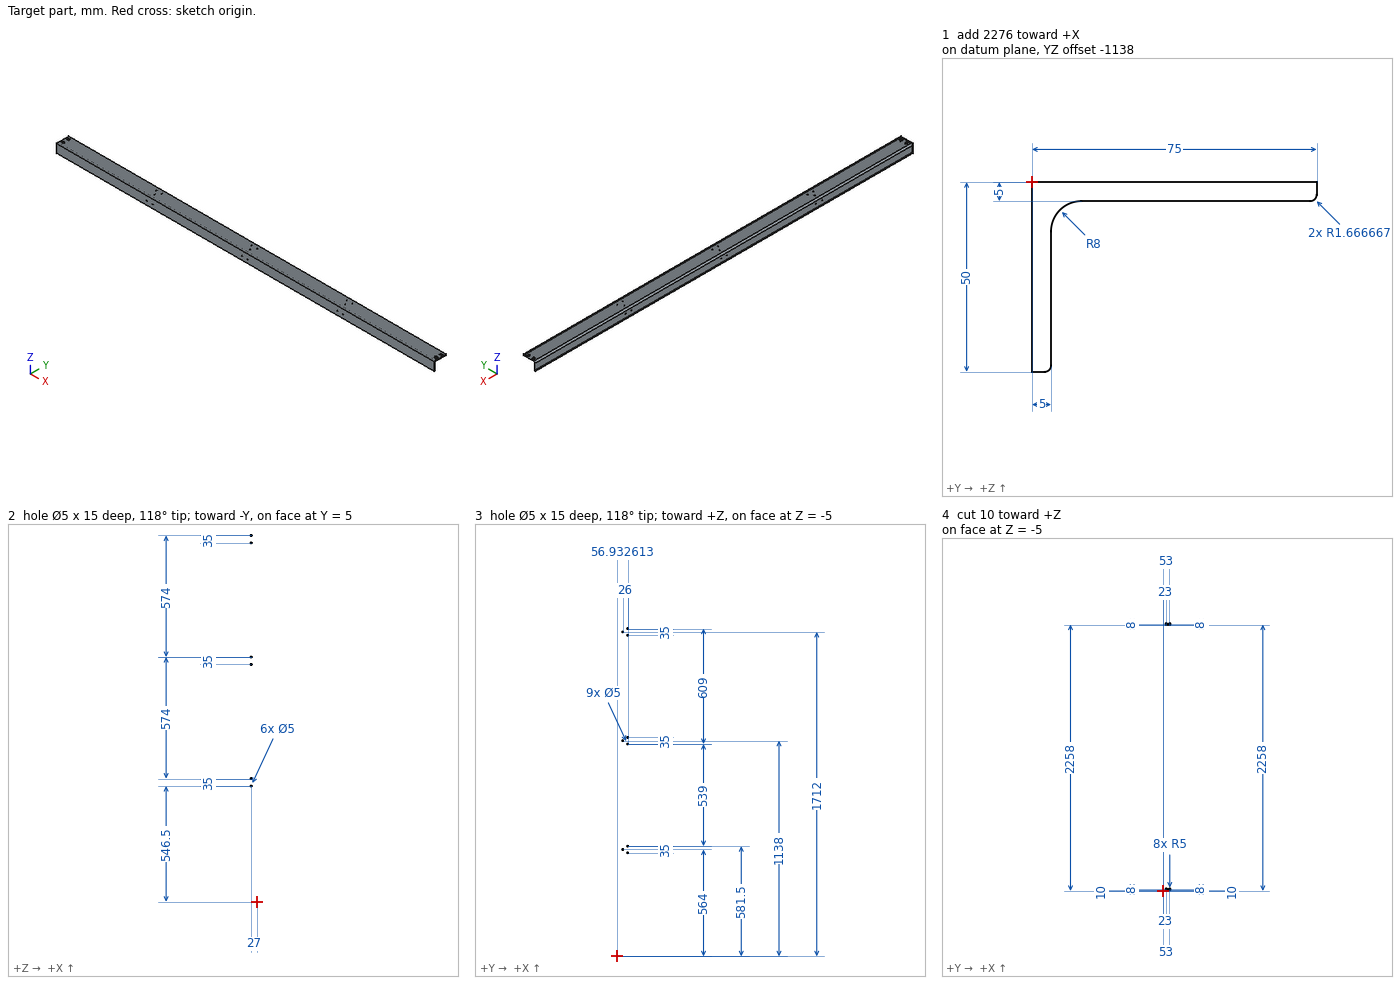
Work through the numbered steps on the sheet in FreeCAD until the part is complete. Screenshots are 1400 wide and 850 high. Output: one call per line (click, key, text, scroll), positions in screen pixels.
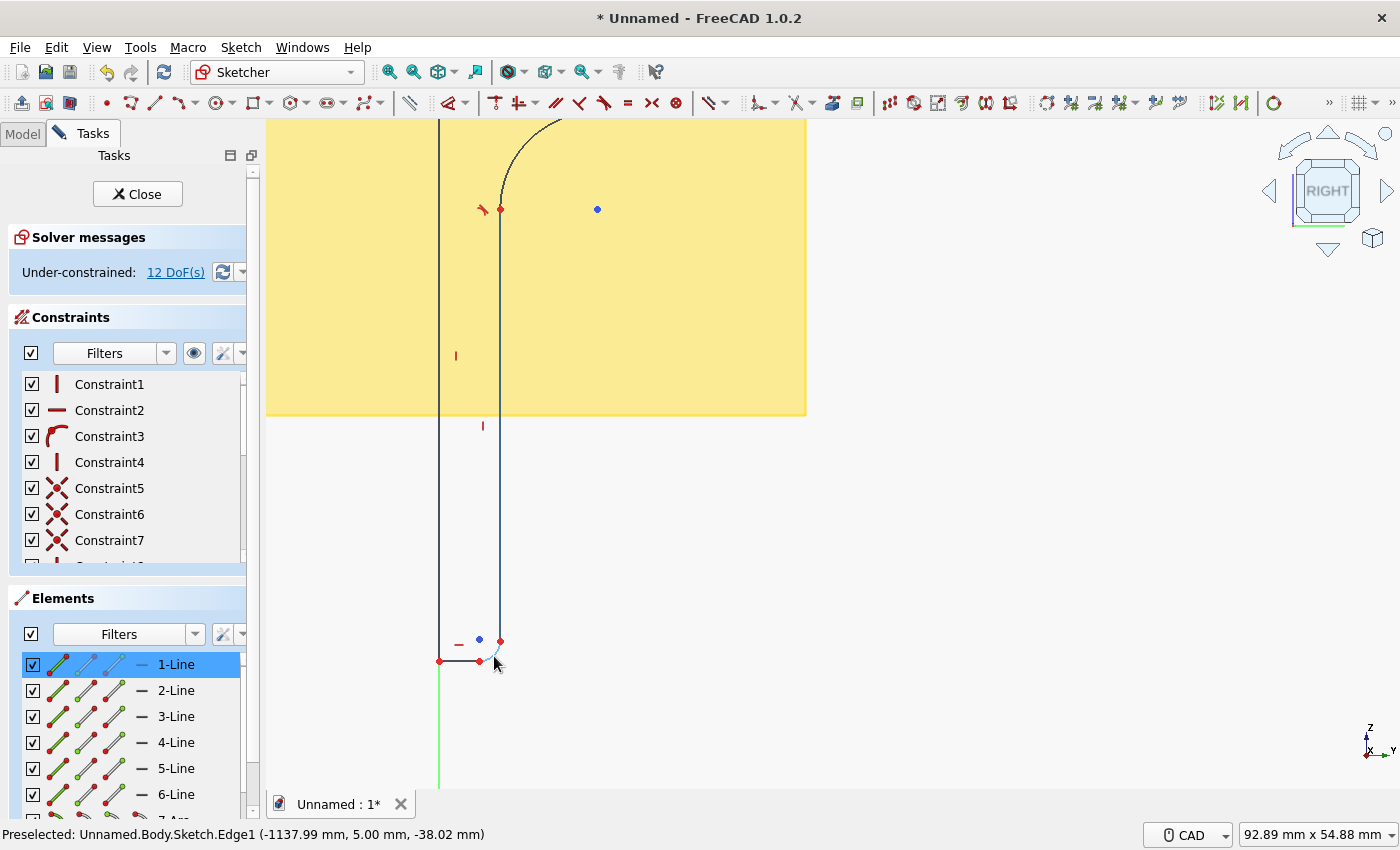
click(494, 656)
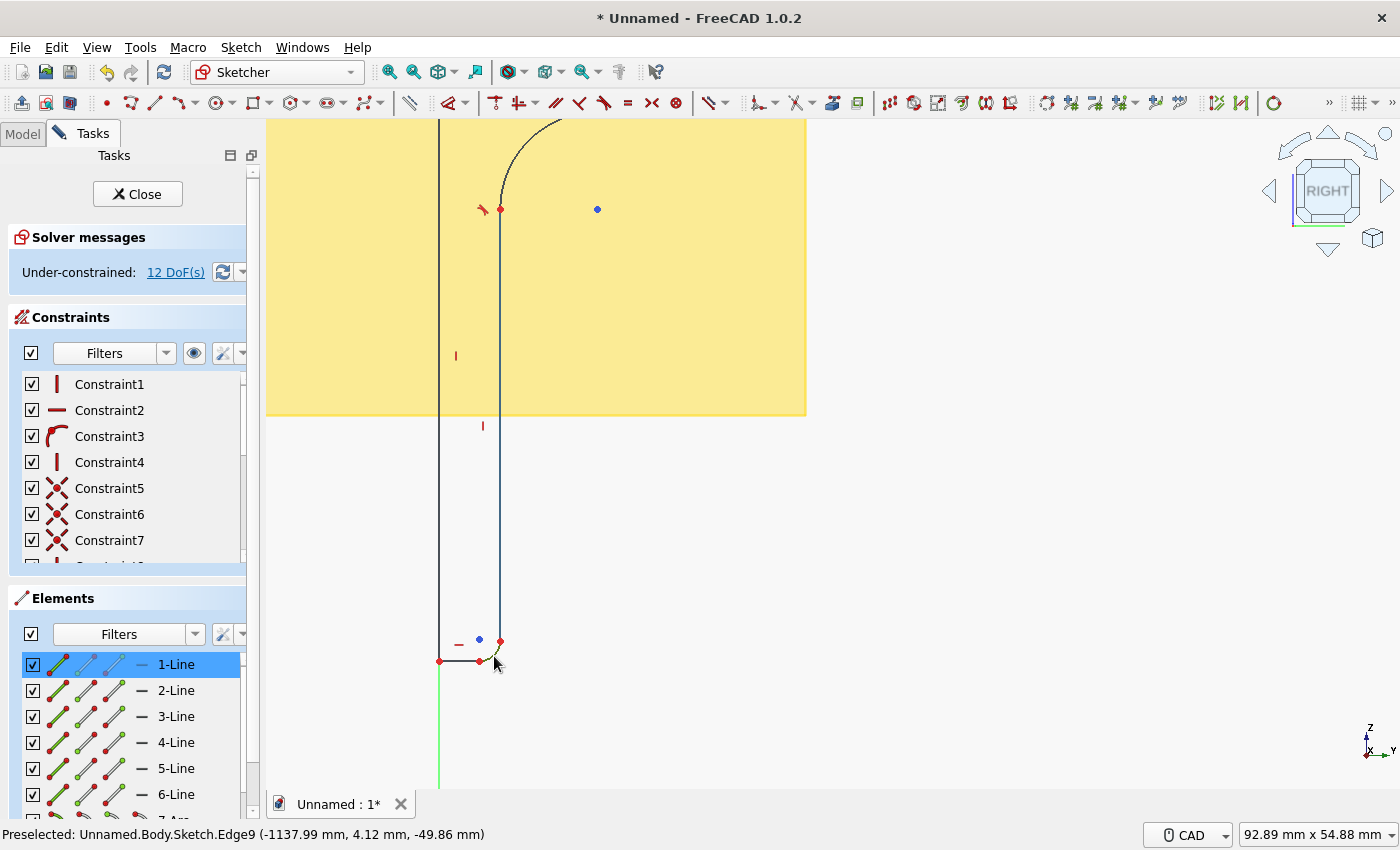
click(604, 104)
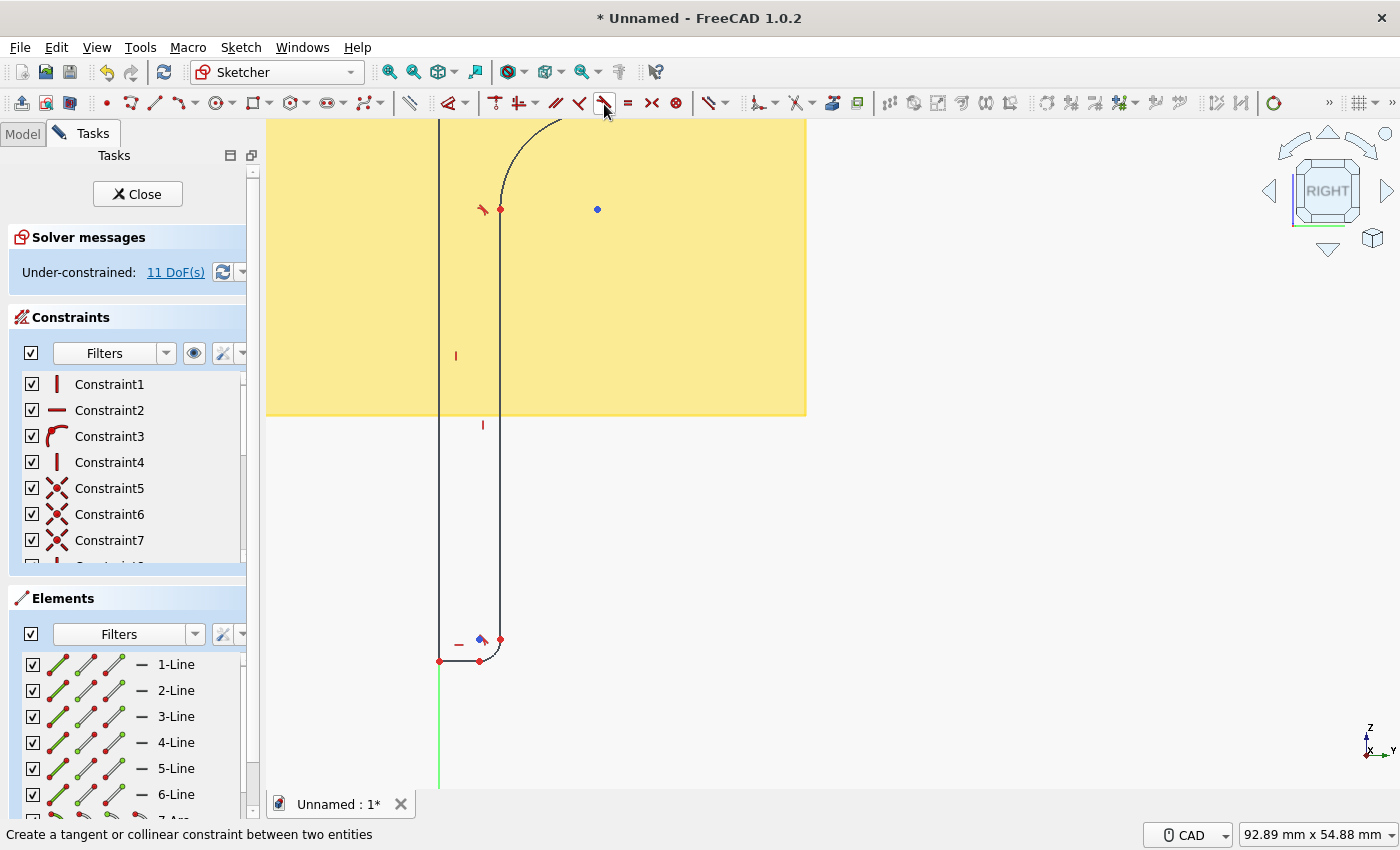
scroll(495, 656, down, 2)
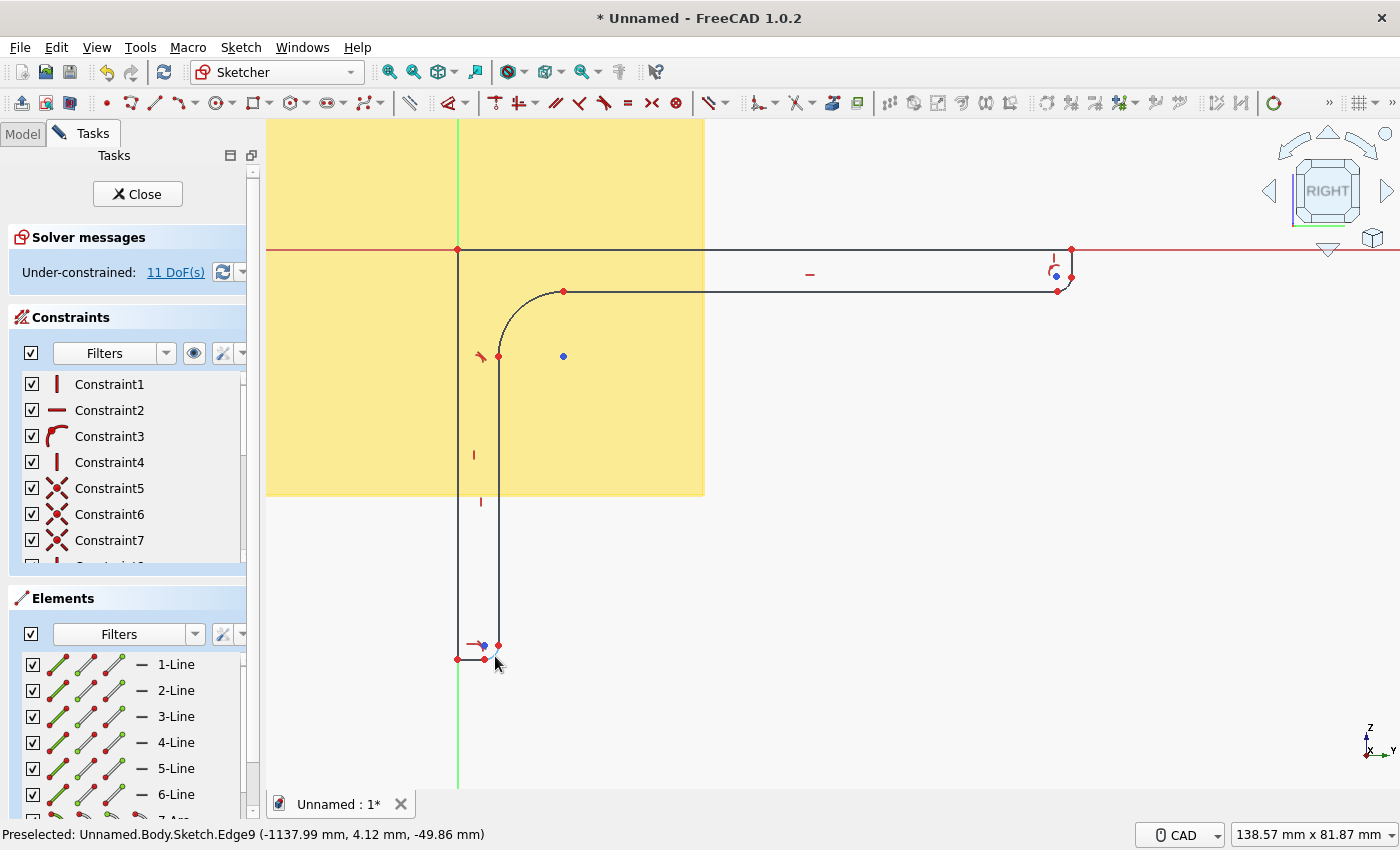
click(712, 292)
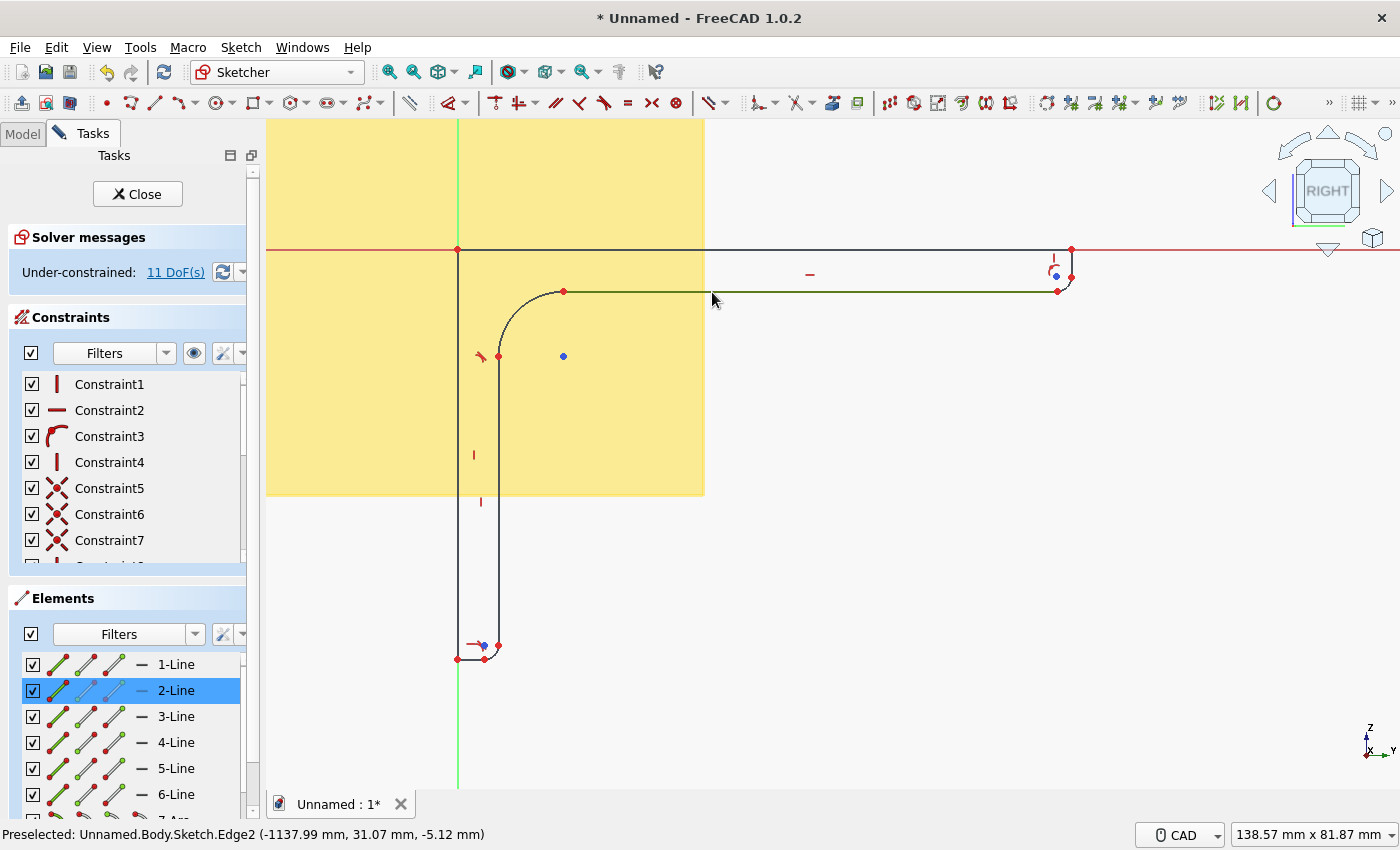
click(534, 299)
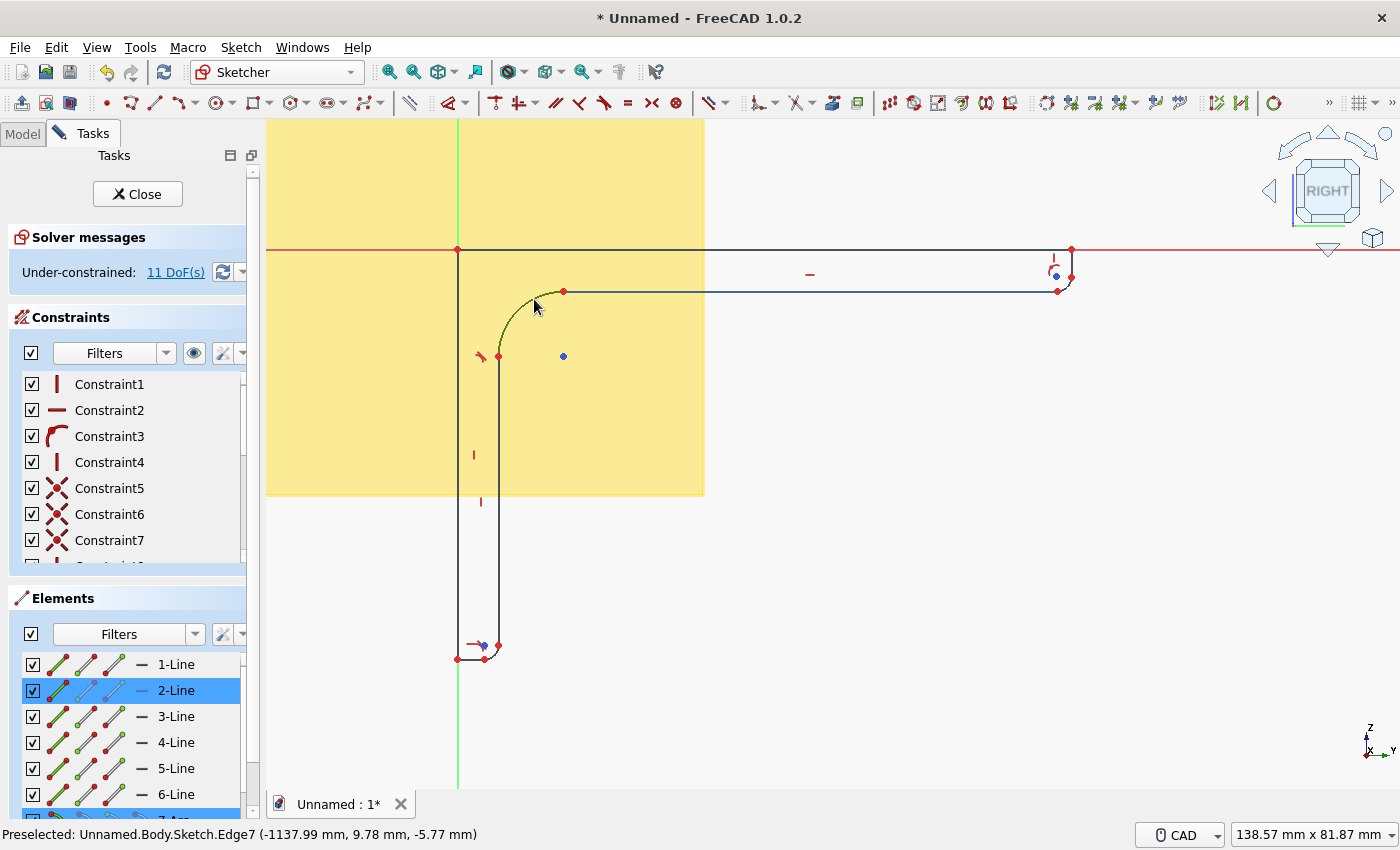
click(604, 104)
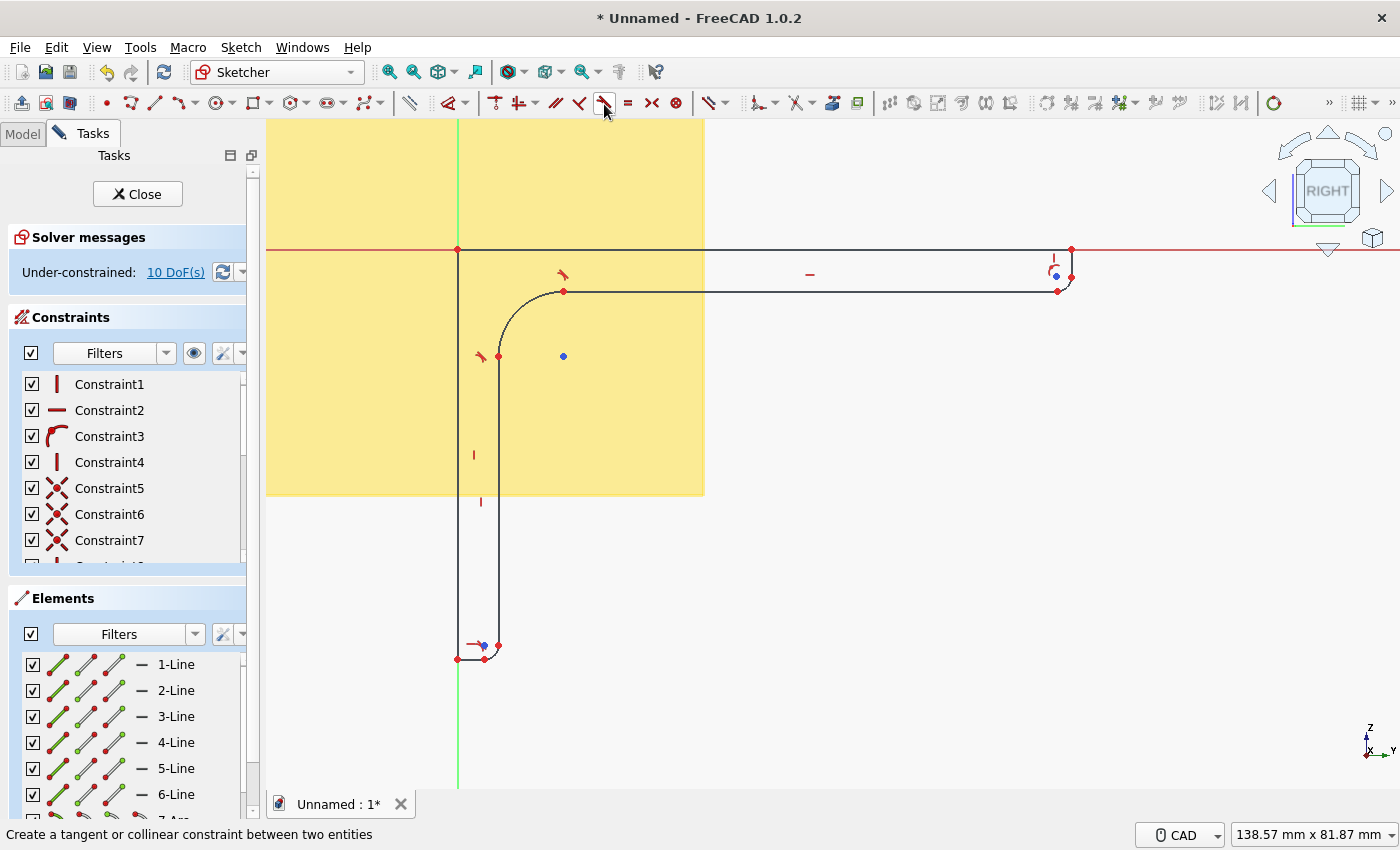
click(712, 292)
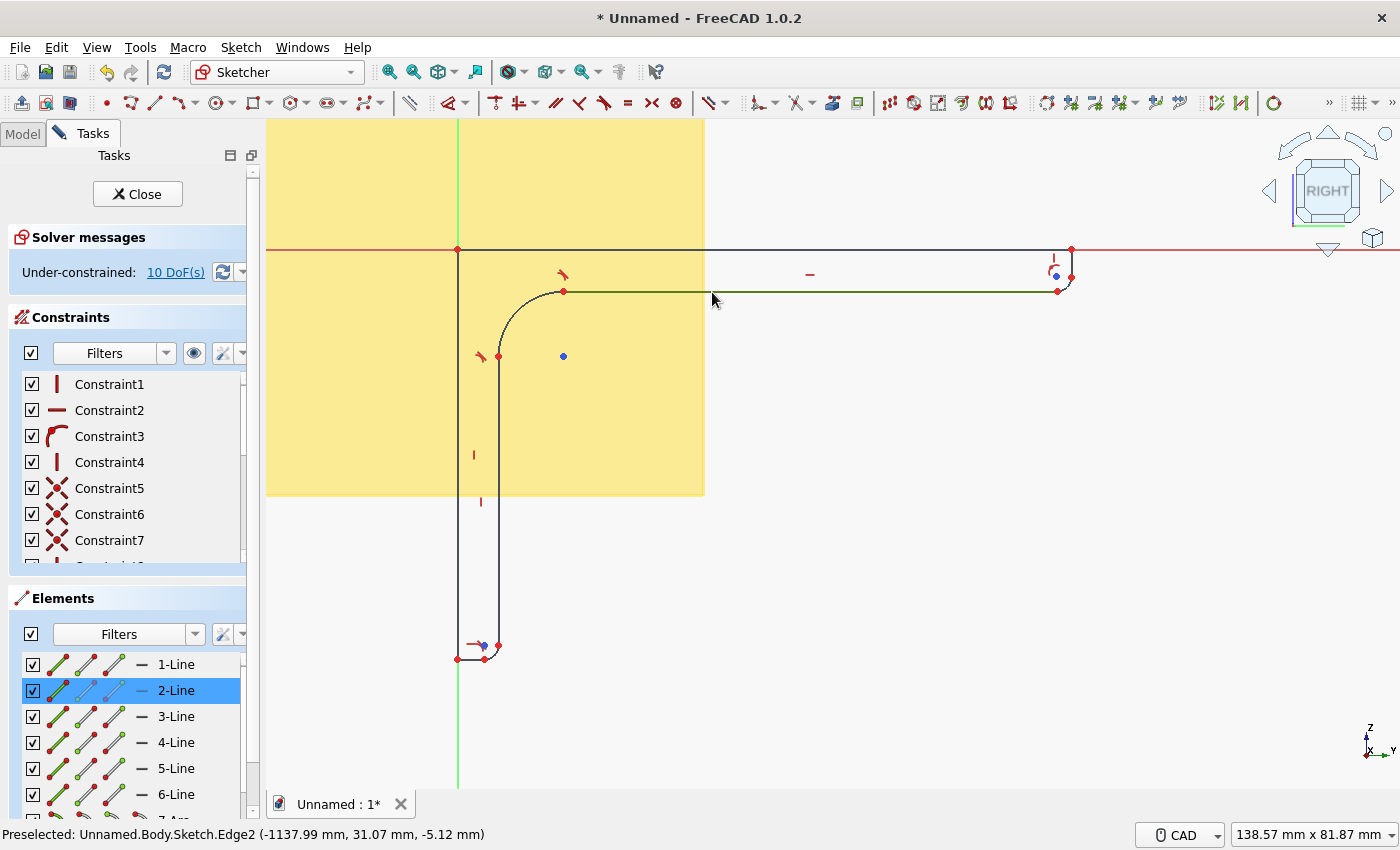
scroll(1067, 287, up, 2)